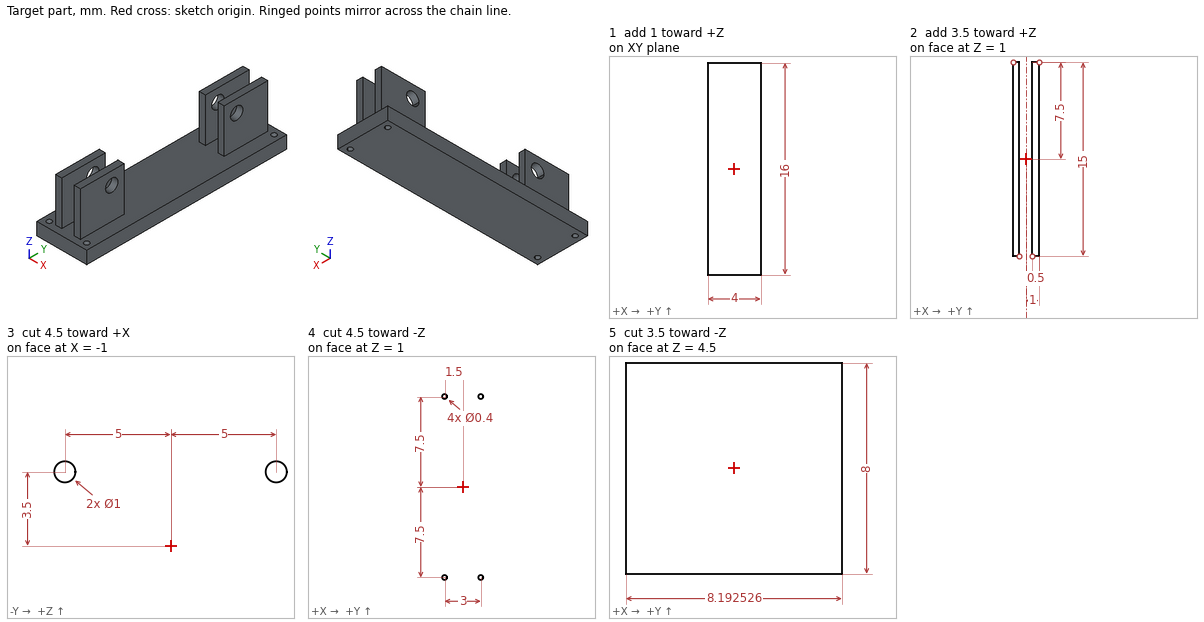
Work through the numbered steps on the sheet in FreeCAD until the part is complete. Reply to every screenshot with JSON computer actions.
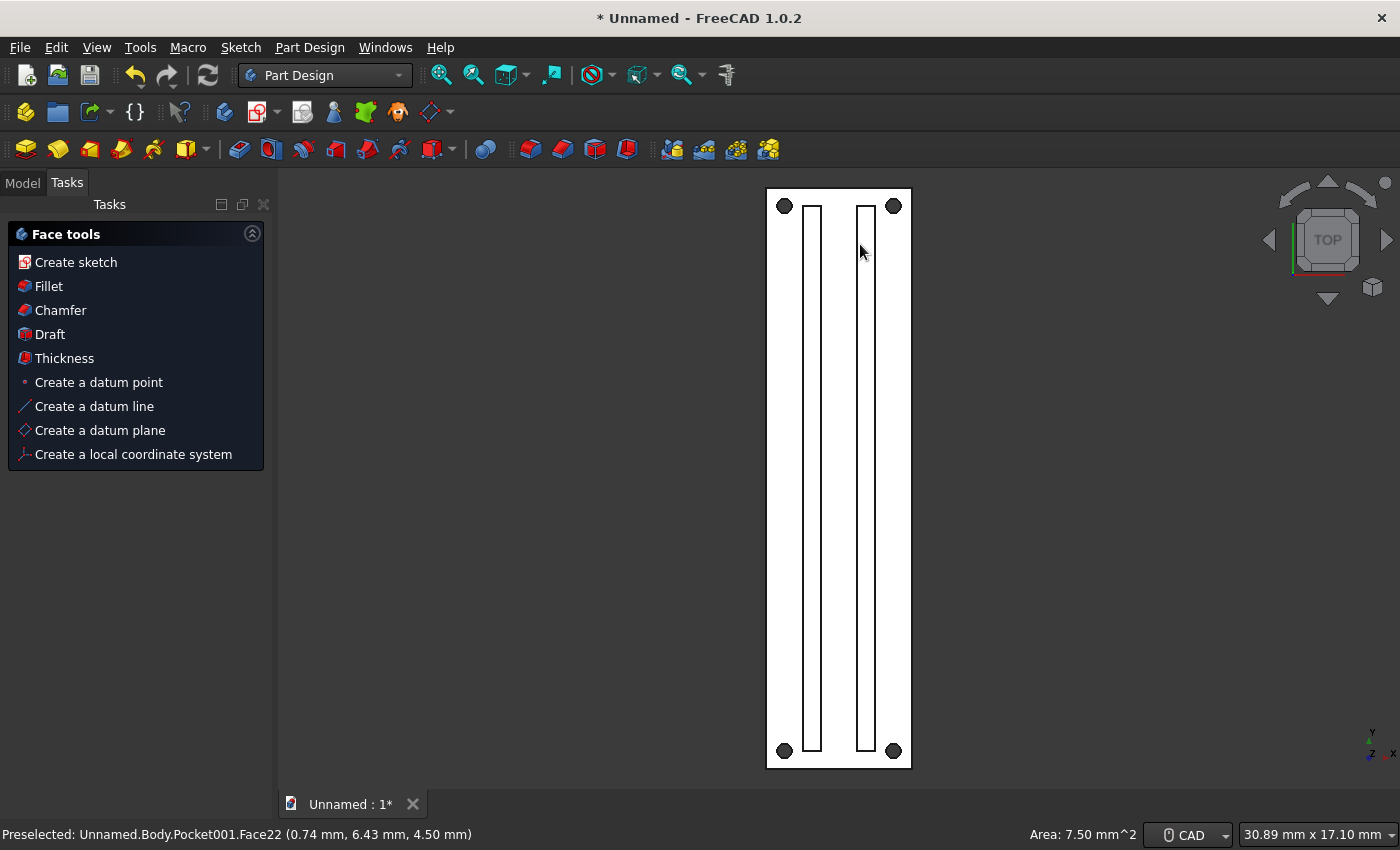
{"action": "left_click", "coordinate": [258, 112]}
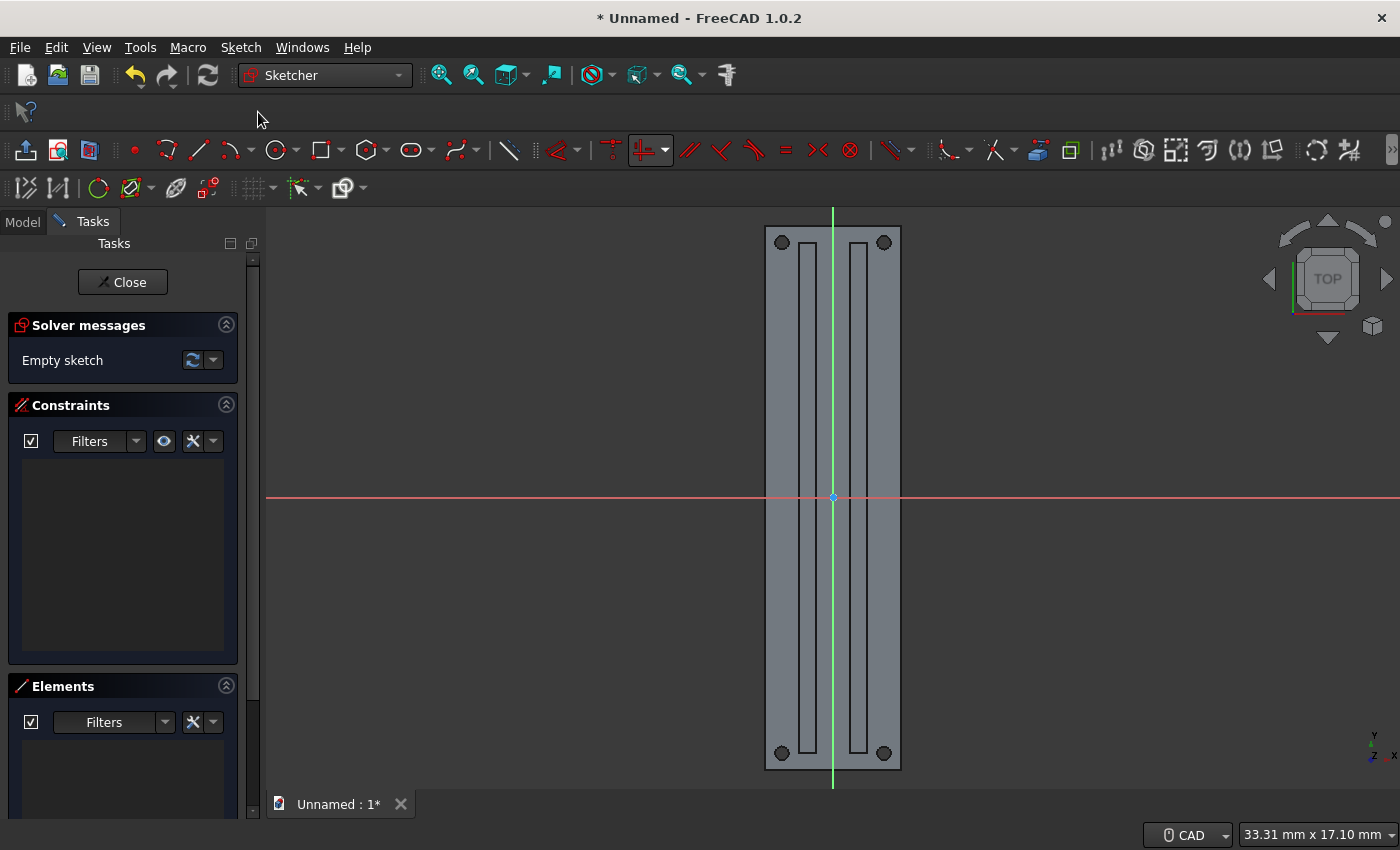
{"action": "scroll", "coordinate": [972, 498], "scroll_direction": "up", "scroll_amount": 2}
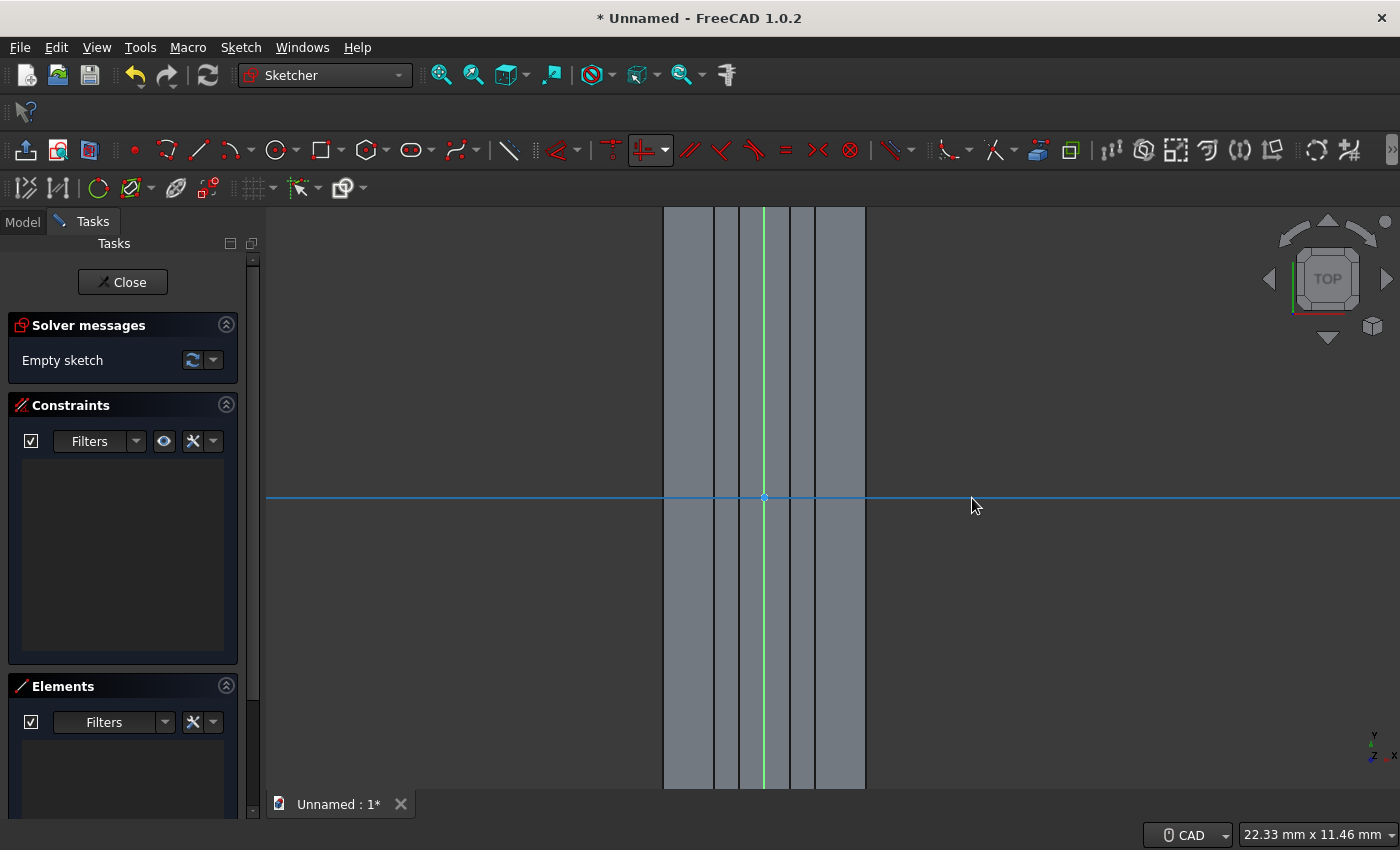
{"action": "key", "text": "g v"}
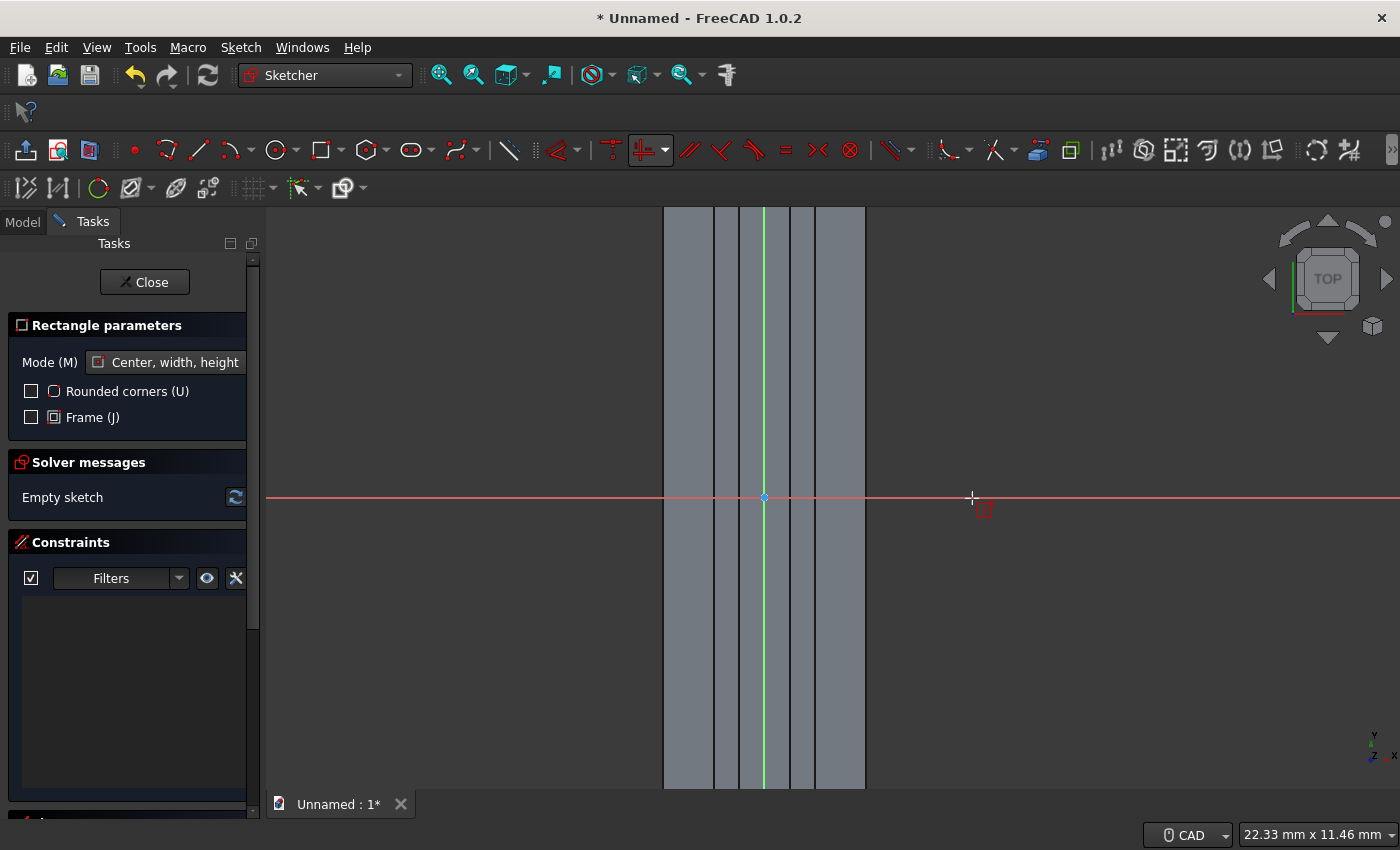
{"action": "left_click", "coordinate": [764, 498]}
{"action": "left_click", "coordinate": [972, 295]}
{"action": "key", "text": "Escape"}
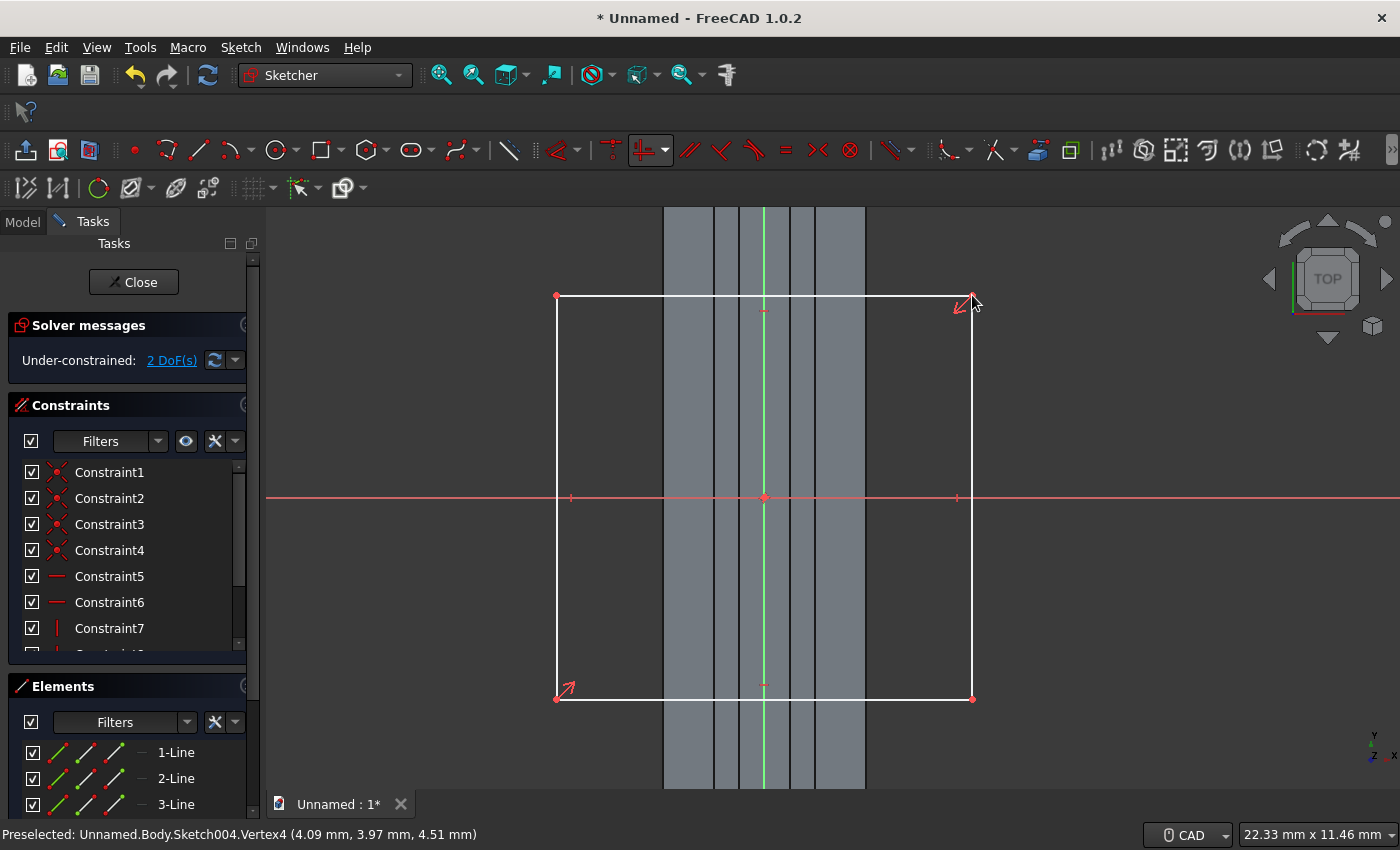
{"action": "left_click", "coordinate": [556, 150]}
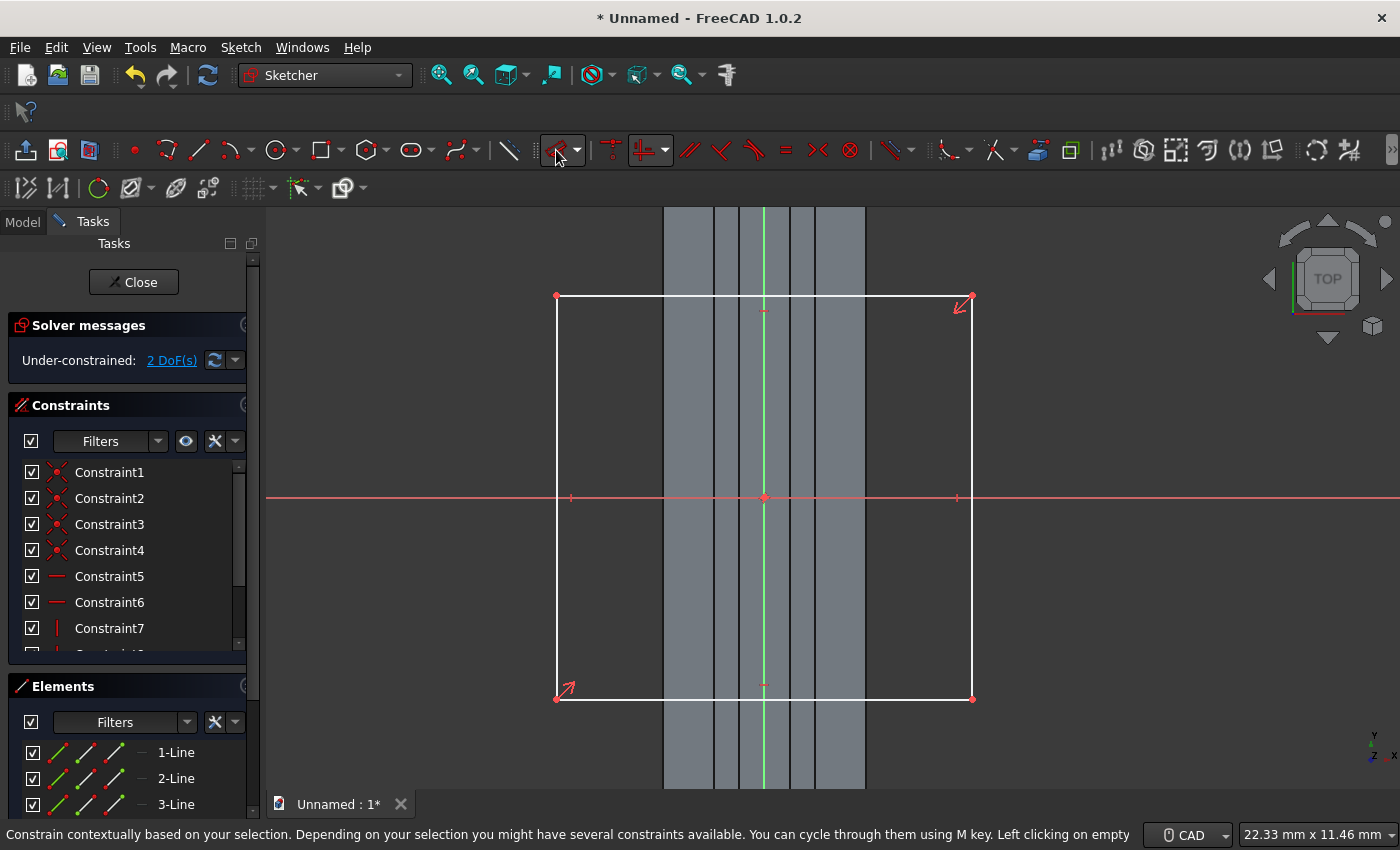
{"action": "left_click", "coordinate": [972, 578]}
{"action": "left_click", "coordinate": [1006, 405]}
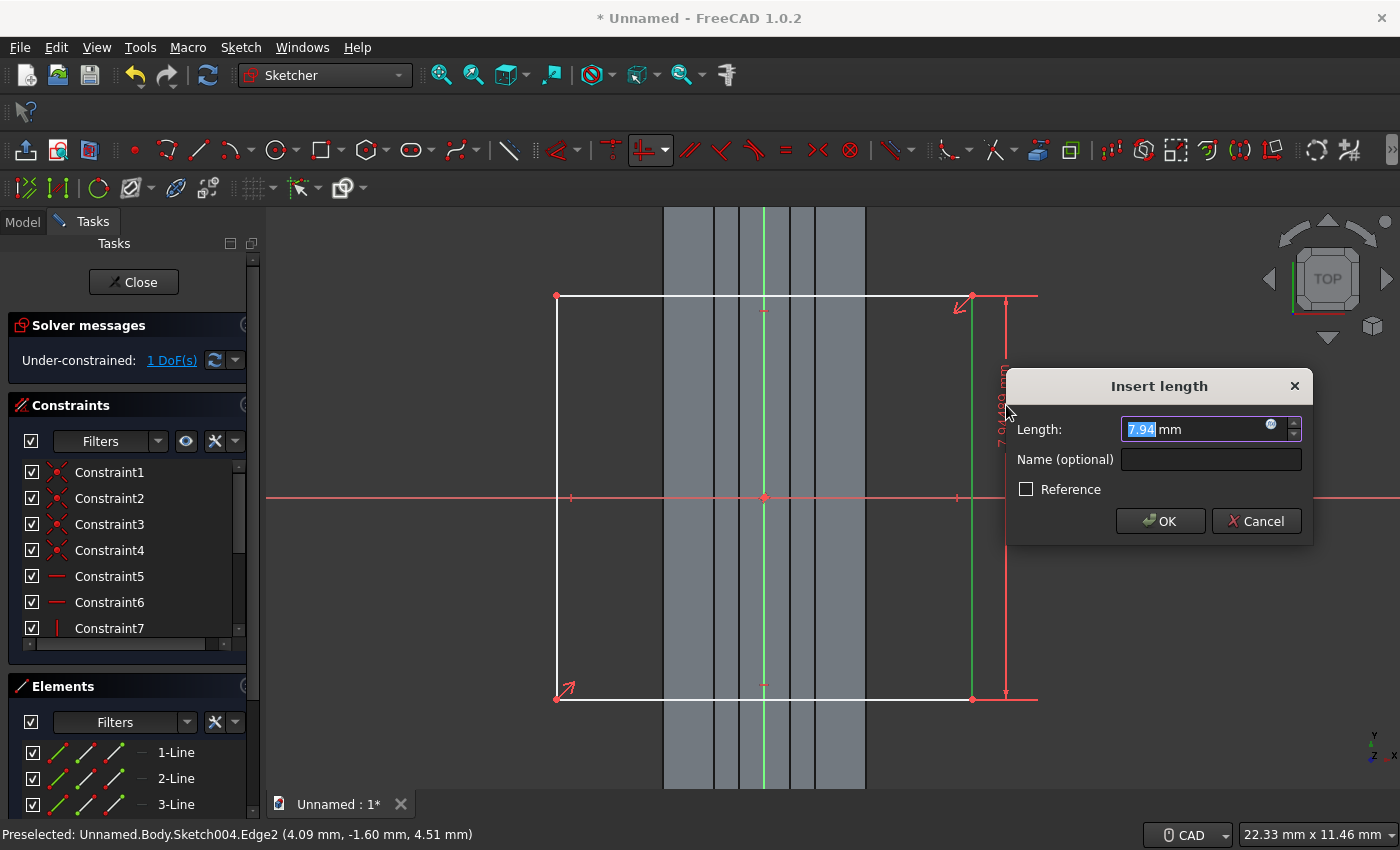
{"action": "type", "text": "8"}
{"action": "key", "text": "Return"}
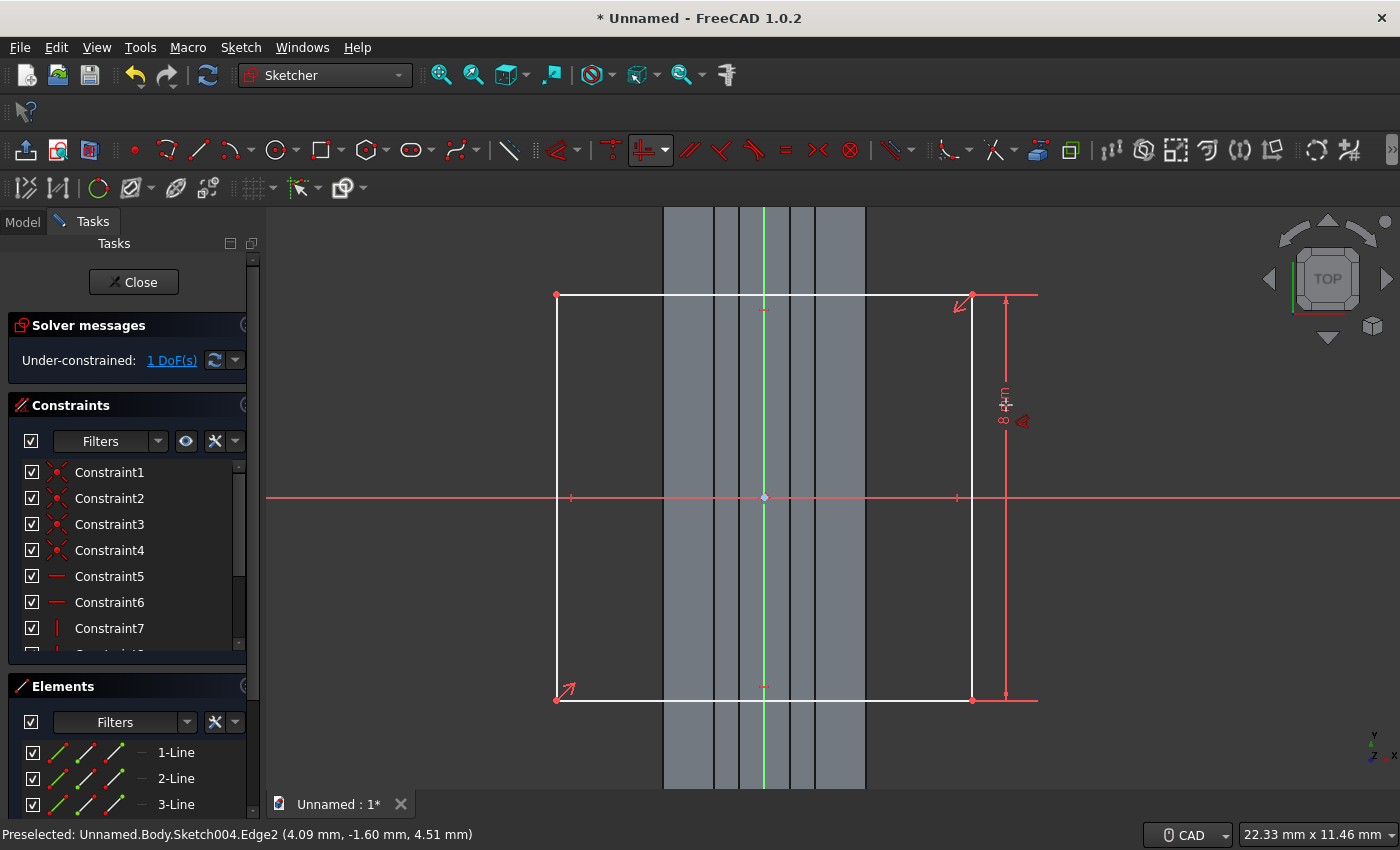
{"action": "left_click", "coordinate": [681, 701]}
{"action": "left_click", "coordinate": [669, 735]}